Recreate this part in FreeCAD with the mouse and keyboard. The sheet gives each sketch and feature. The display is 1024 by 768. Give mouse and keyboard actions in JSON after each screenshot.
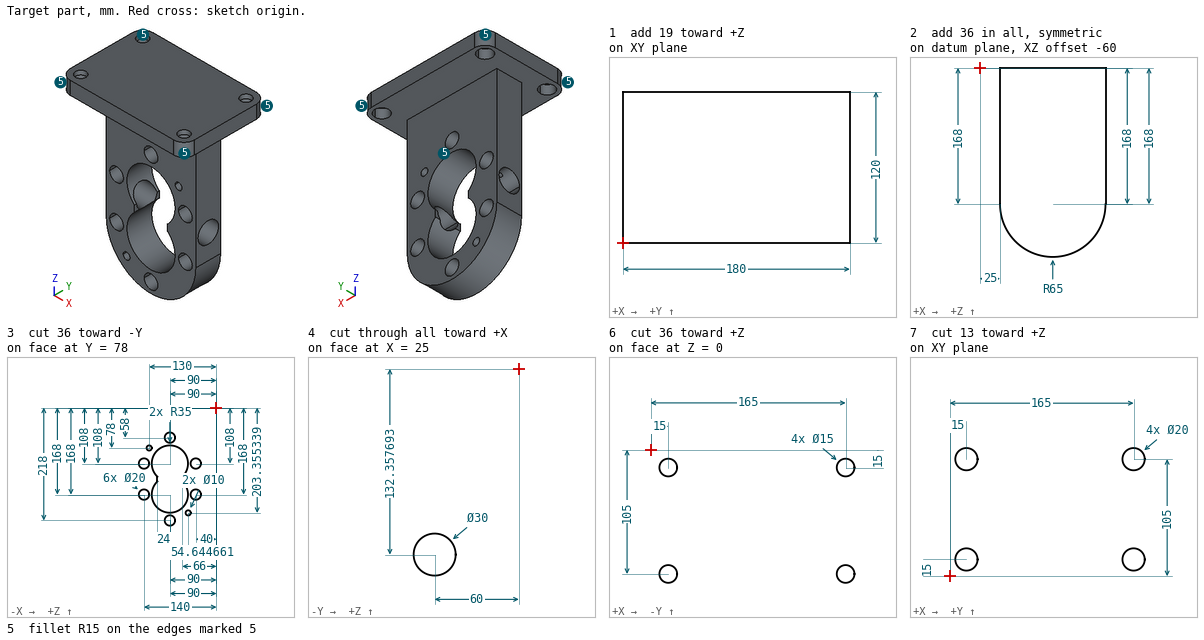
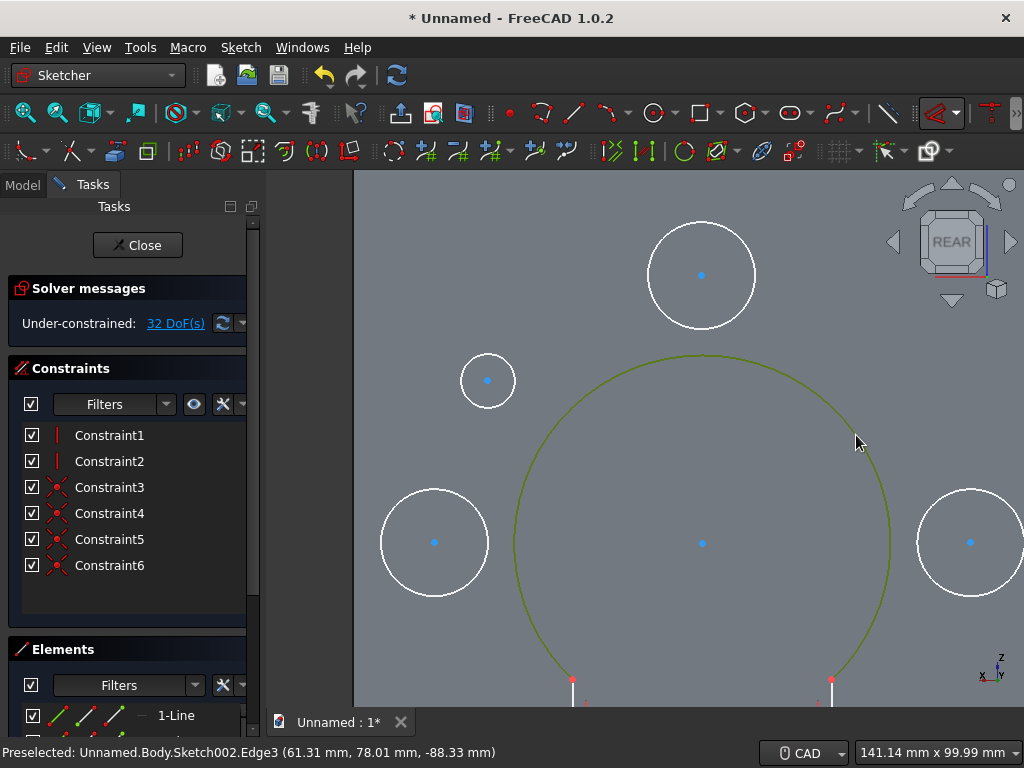
{"action": "scroll", "coordinate": [488, 380], "scroll_direction": "down", "scroll_amount": 6}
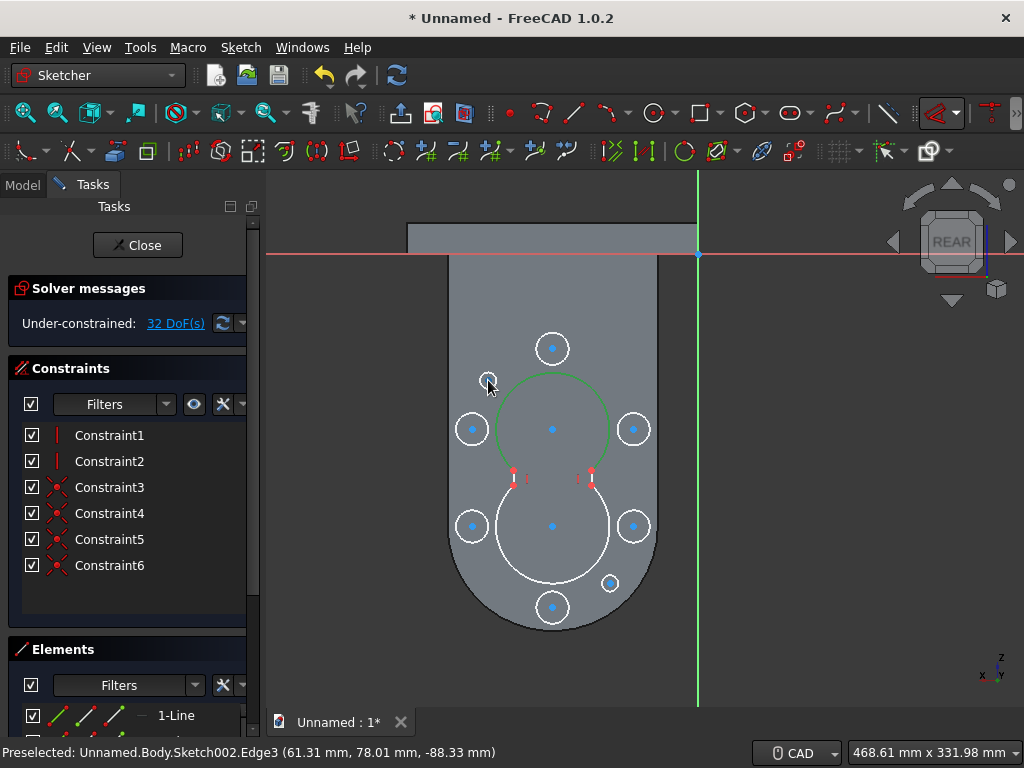
{"action": "left_click", "coordinate": [506, 560]}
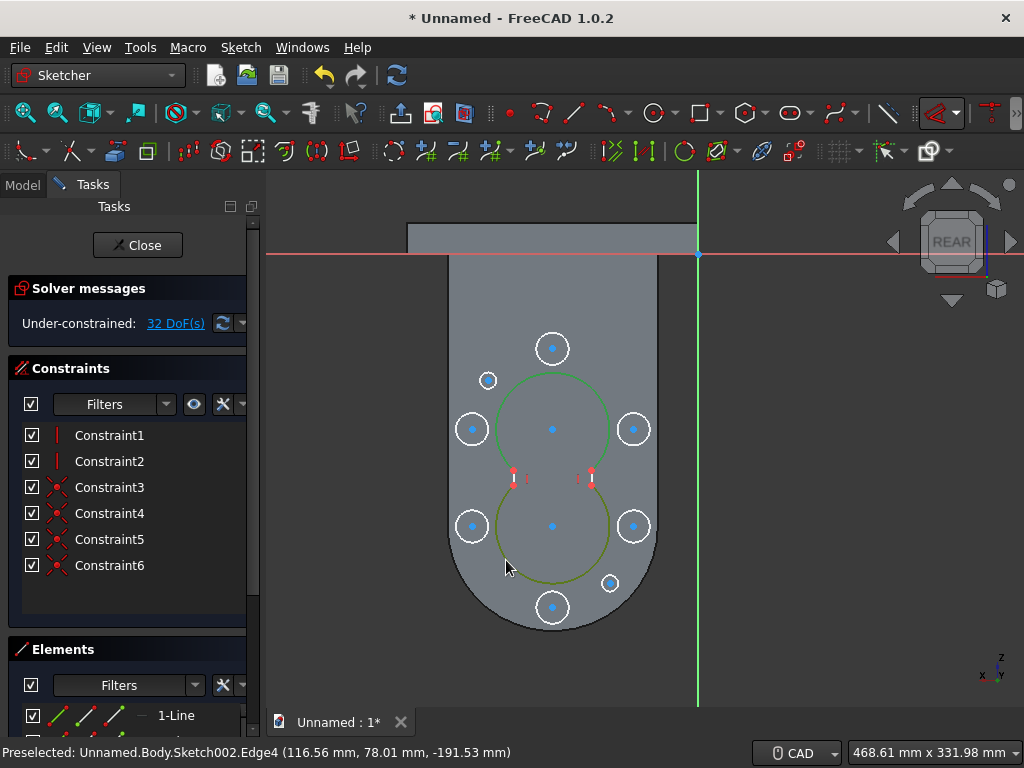
{"action": "key", "text": "e"}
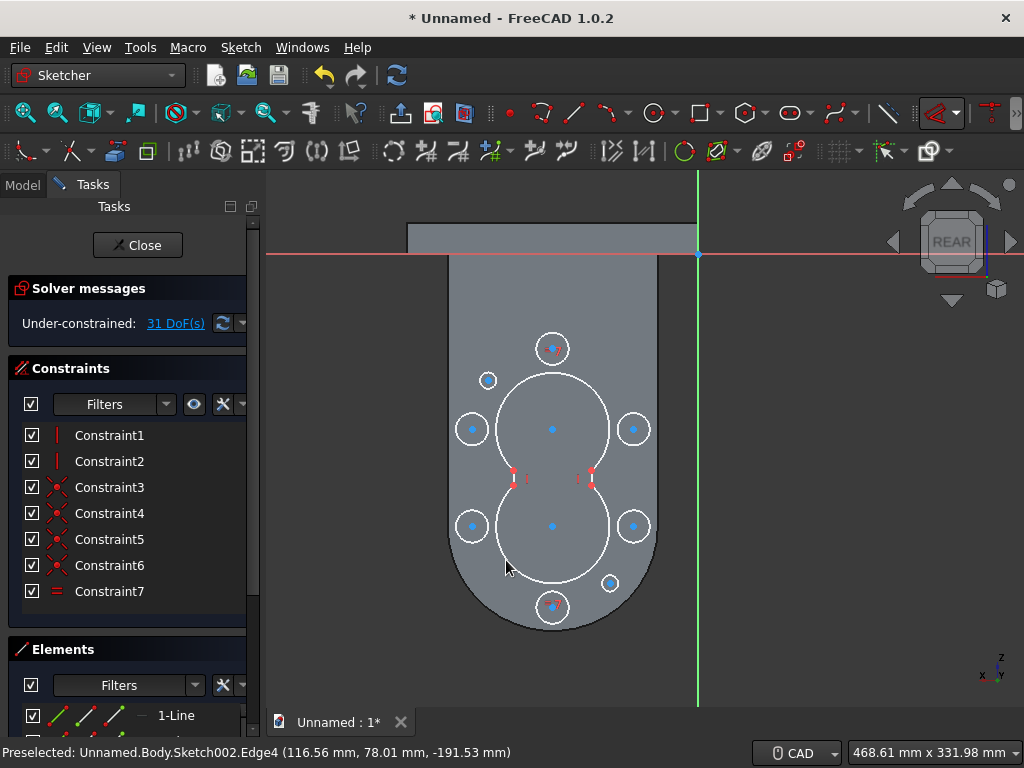
{"action": "left_click", "coordinate": [564, 596]}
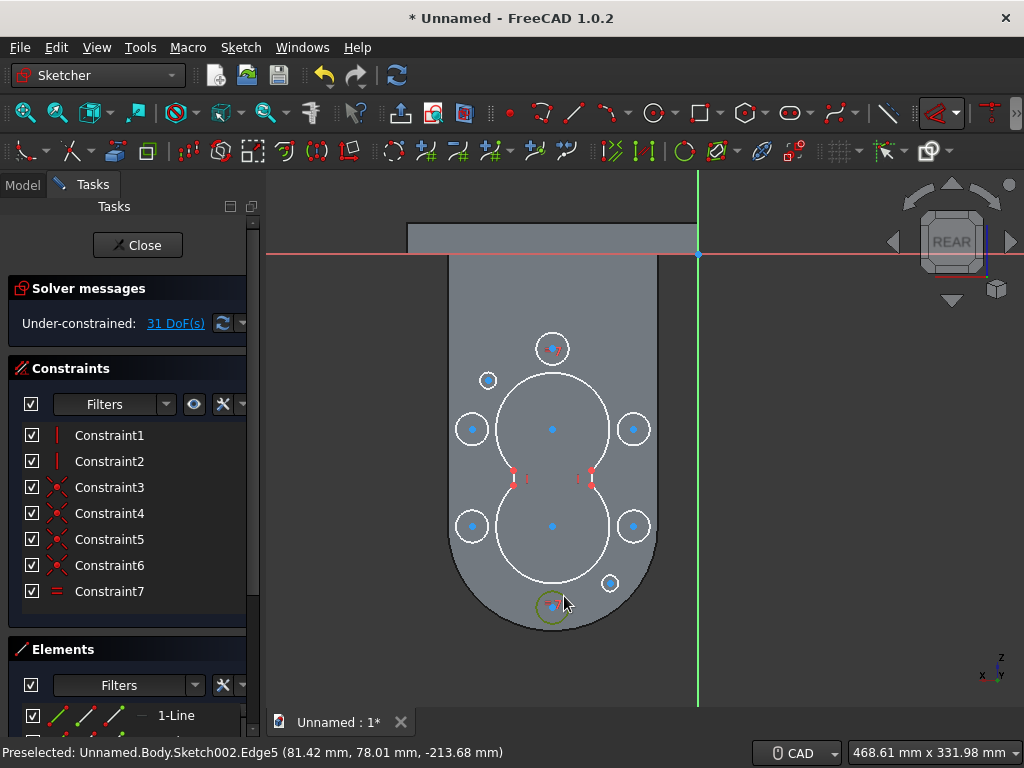
{"action": "left_click", "coordinate": [483, 515]}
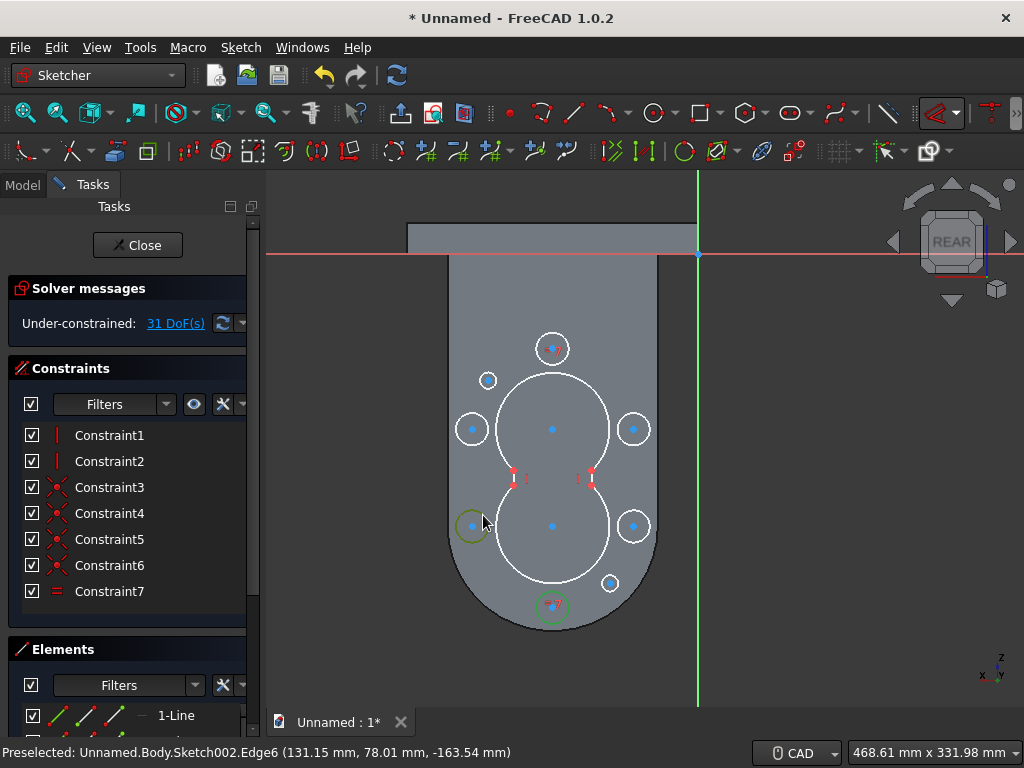
{"action": "left_click", "coordinate": [645, 515]}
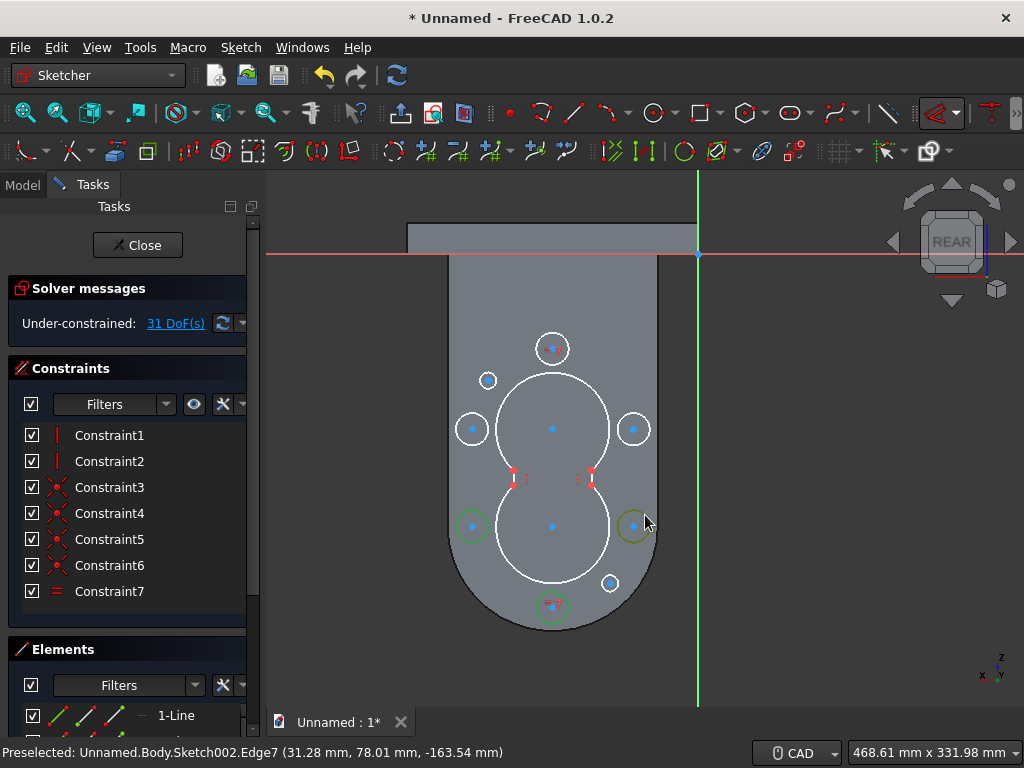
{"action": "left_click", "coordinate": [564, 337]}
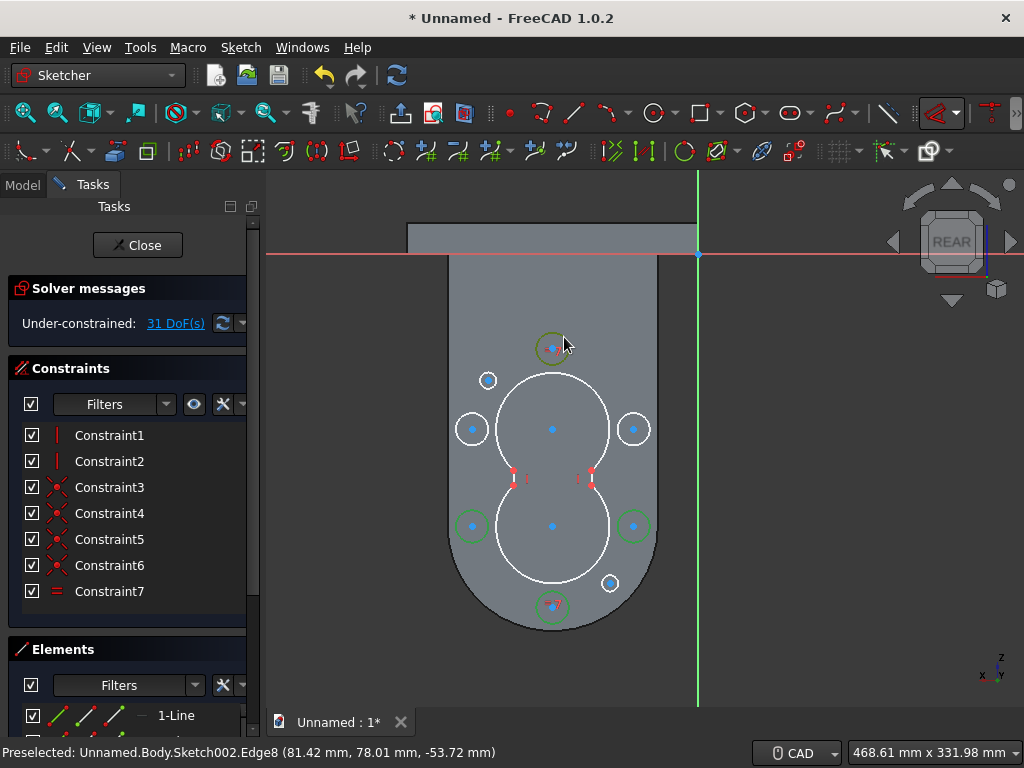
{"action": "left_click", "coordinate": [645, 418]}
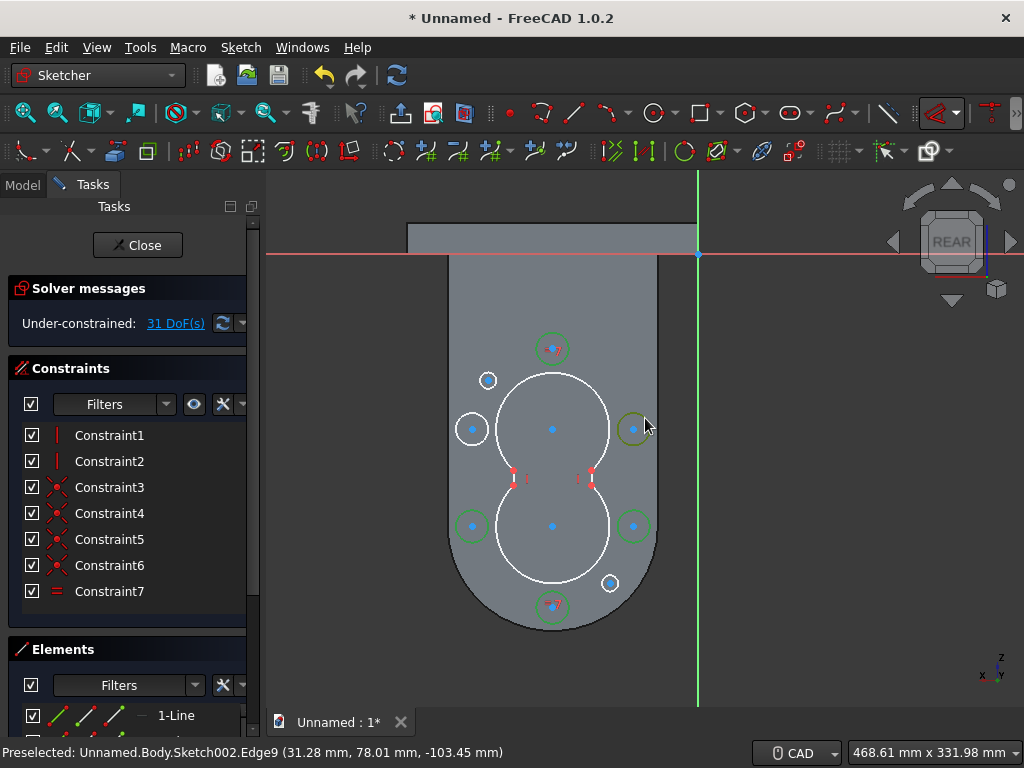
{"action": "left_click", "coordinate": [483, 418]}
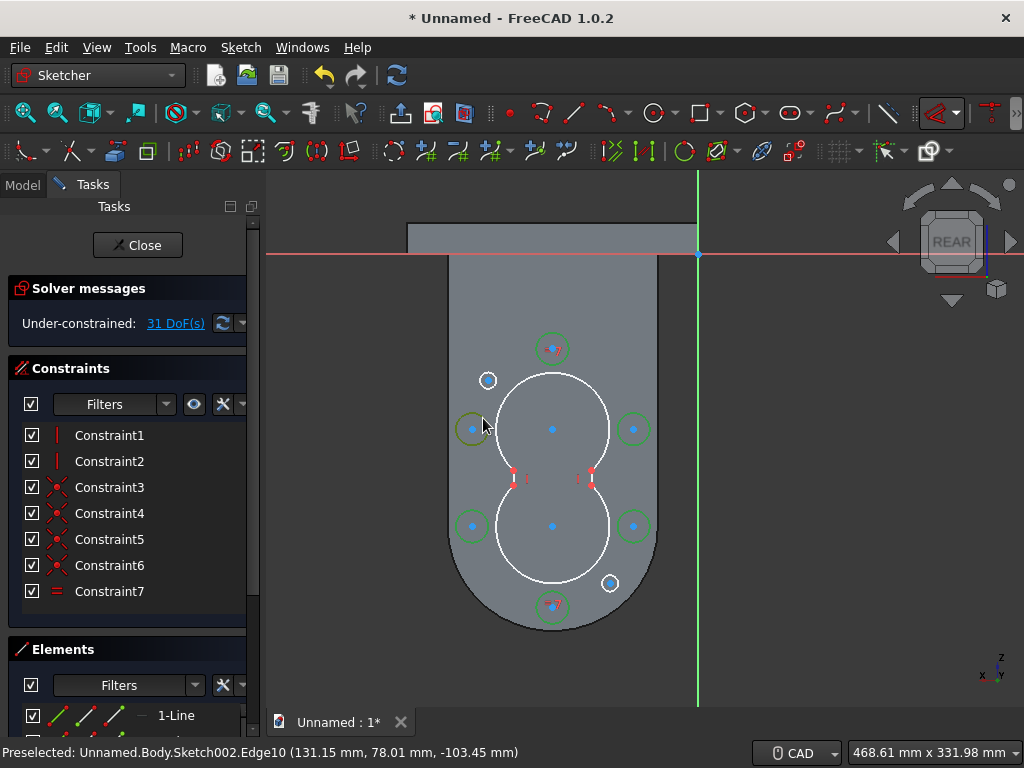
{"action": "key", "text": "e"}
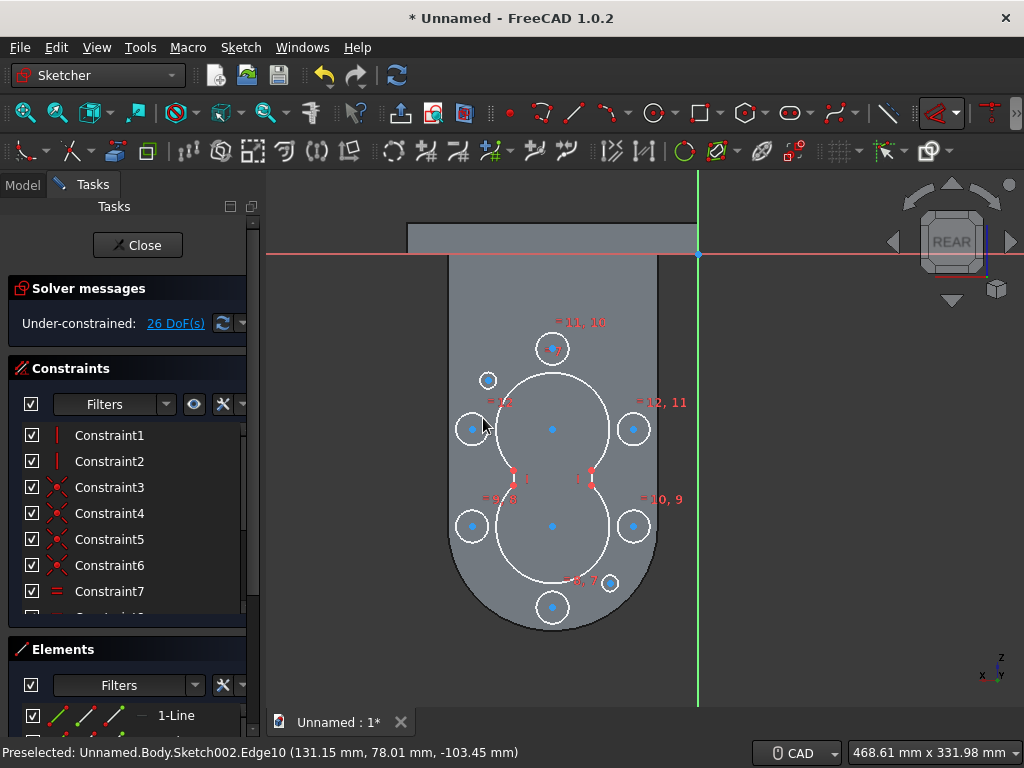
{"action": "scroll", "coordinate": [610, 575], "scroll_direction": "up", "scroll_amount": 3}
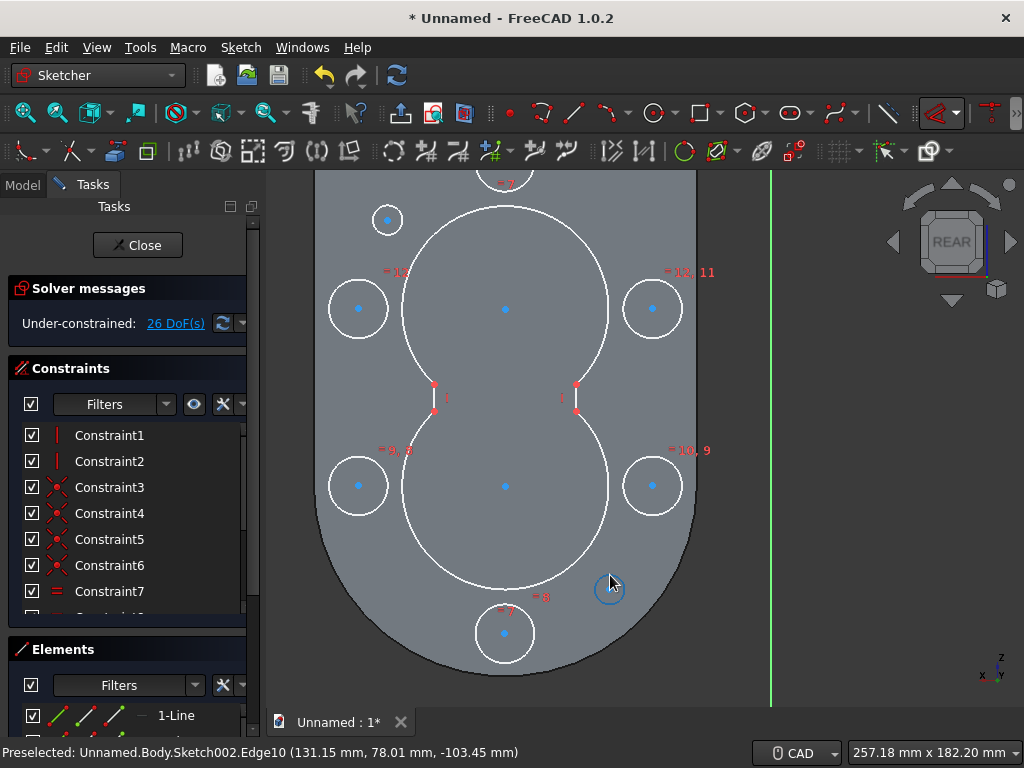
{"action": "left_click", "coordinate": [610, 575]}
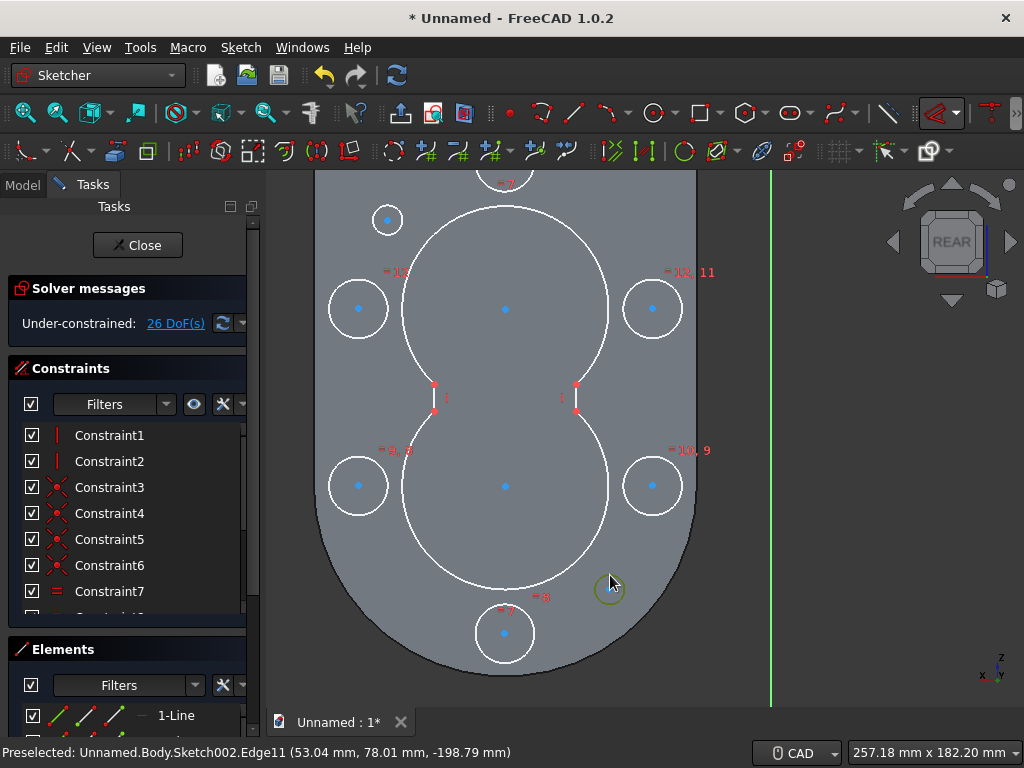
{"action": "left_click", "coordinate": [398, 210]}